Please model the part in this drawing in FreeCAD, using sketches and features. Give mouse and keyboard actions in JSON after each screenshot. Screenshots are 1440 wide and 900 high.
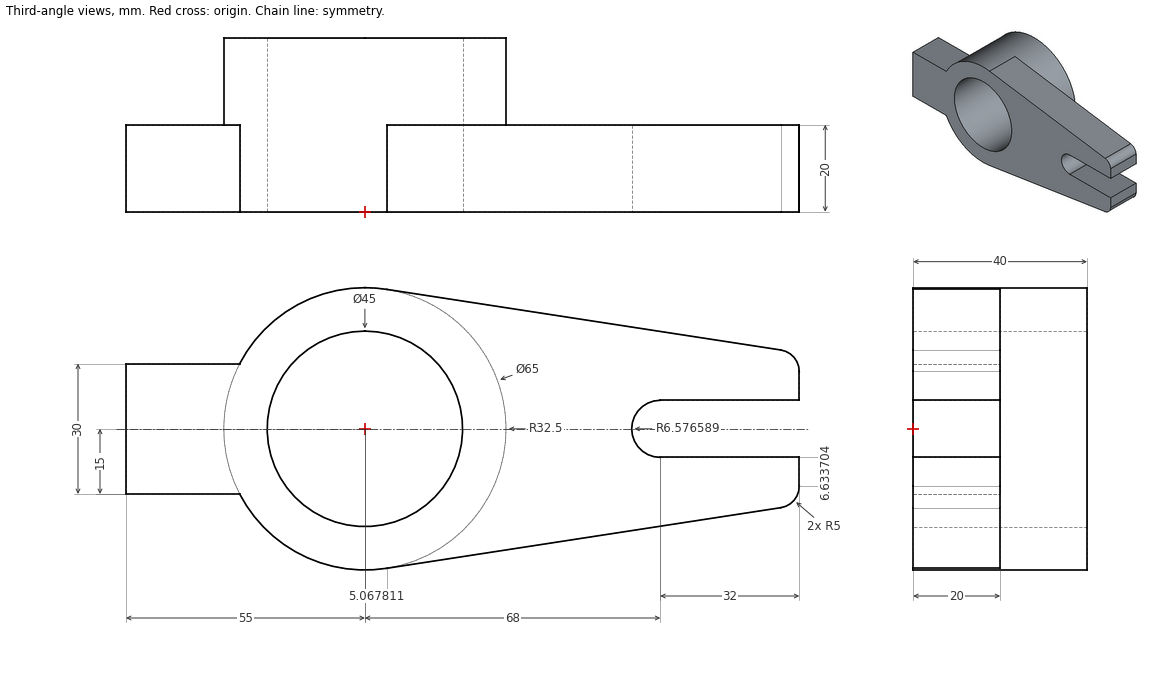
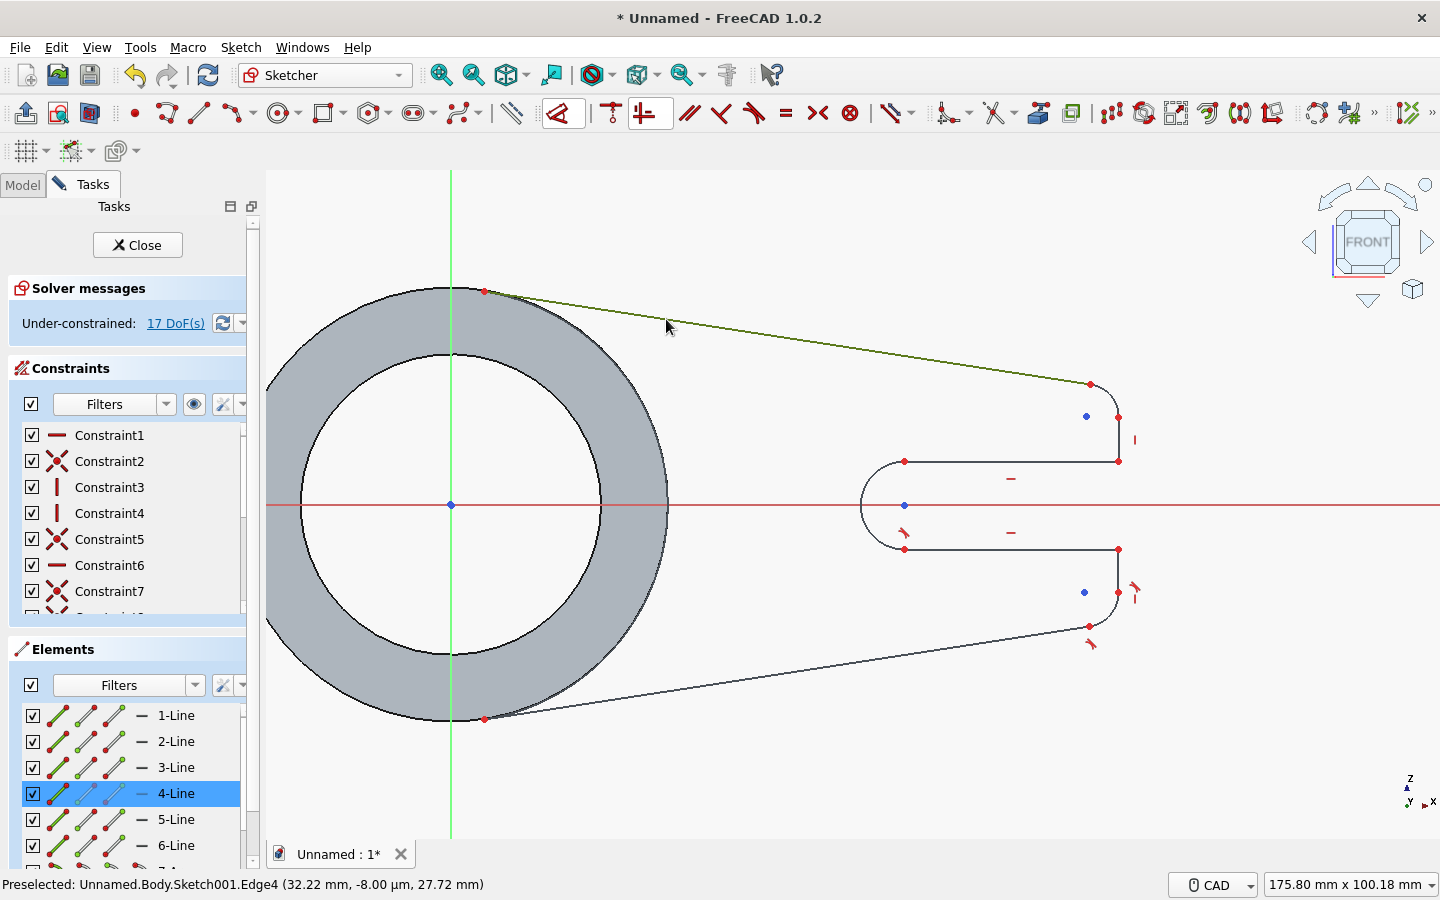
{"action": "left_click", "coordinate": [1116, 404]}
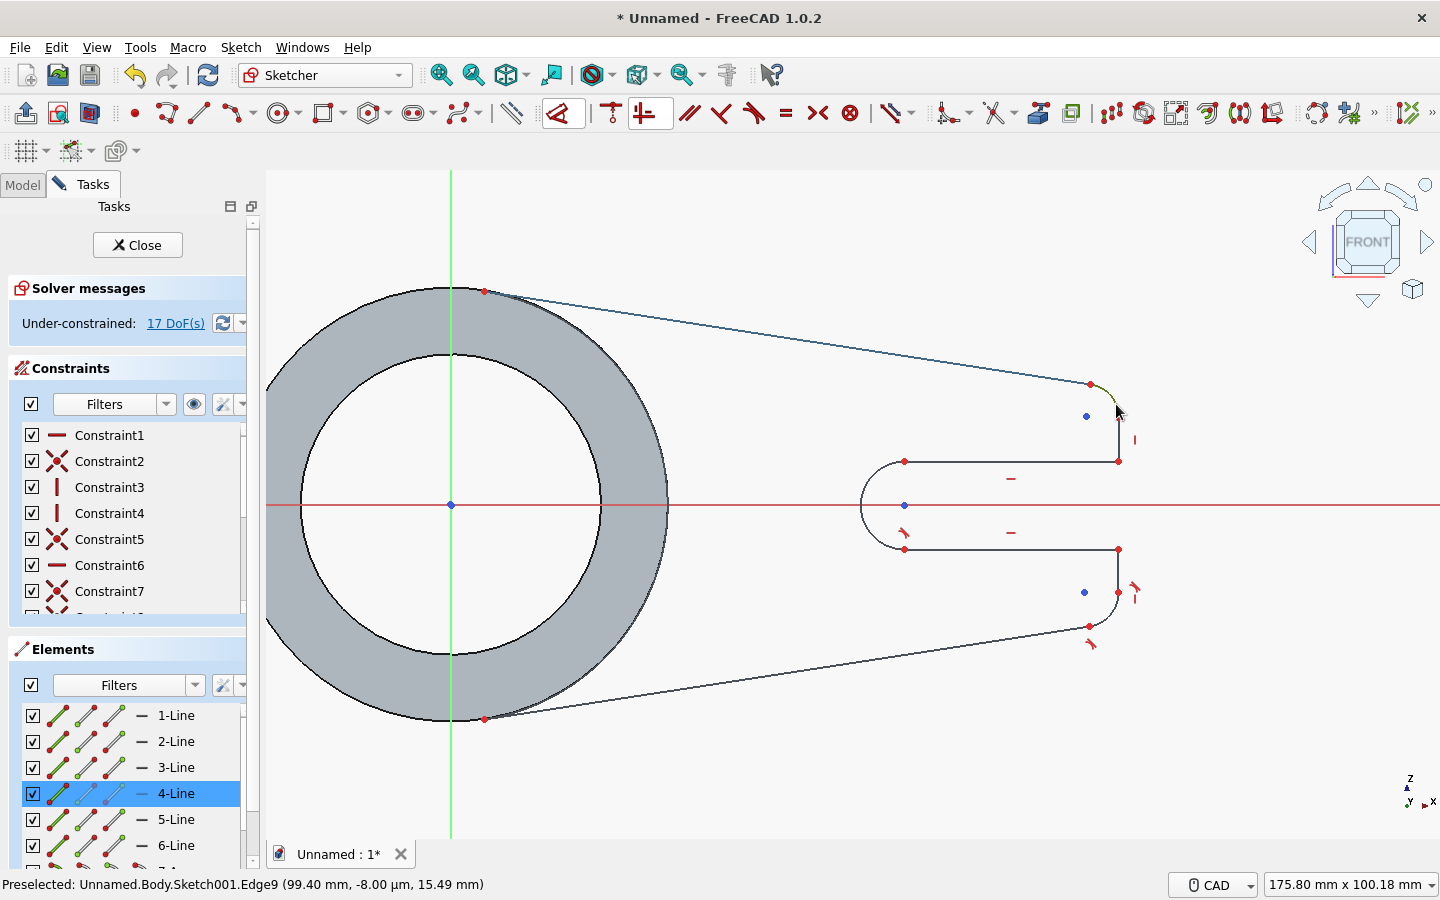
{"action": "left_click", "coordinate": [754, 114]}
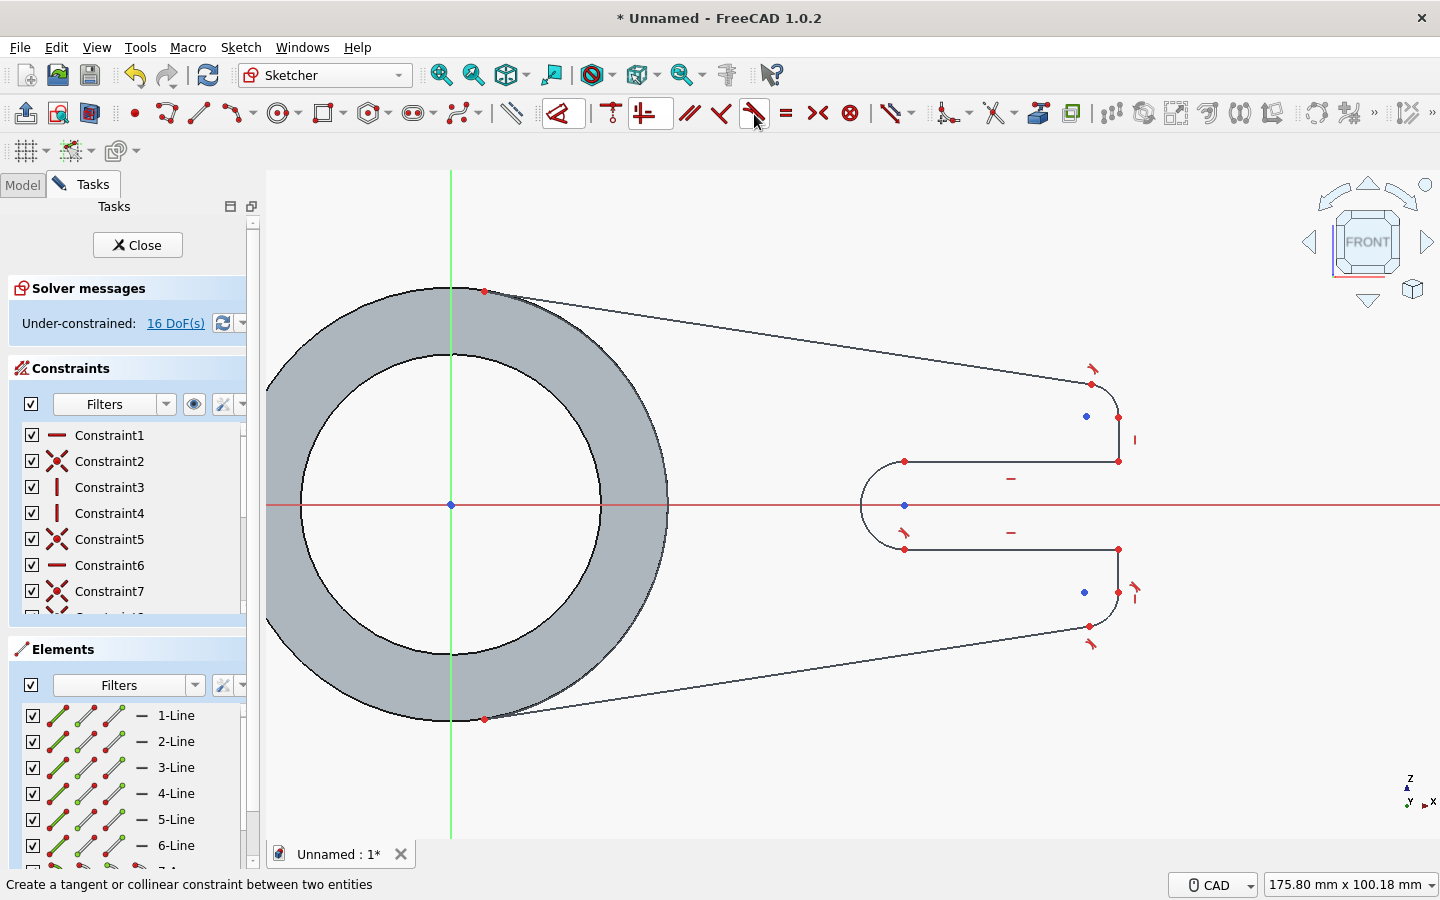
{"action": "left_click", "coordinate": [1119, 431]}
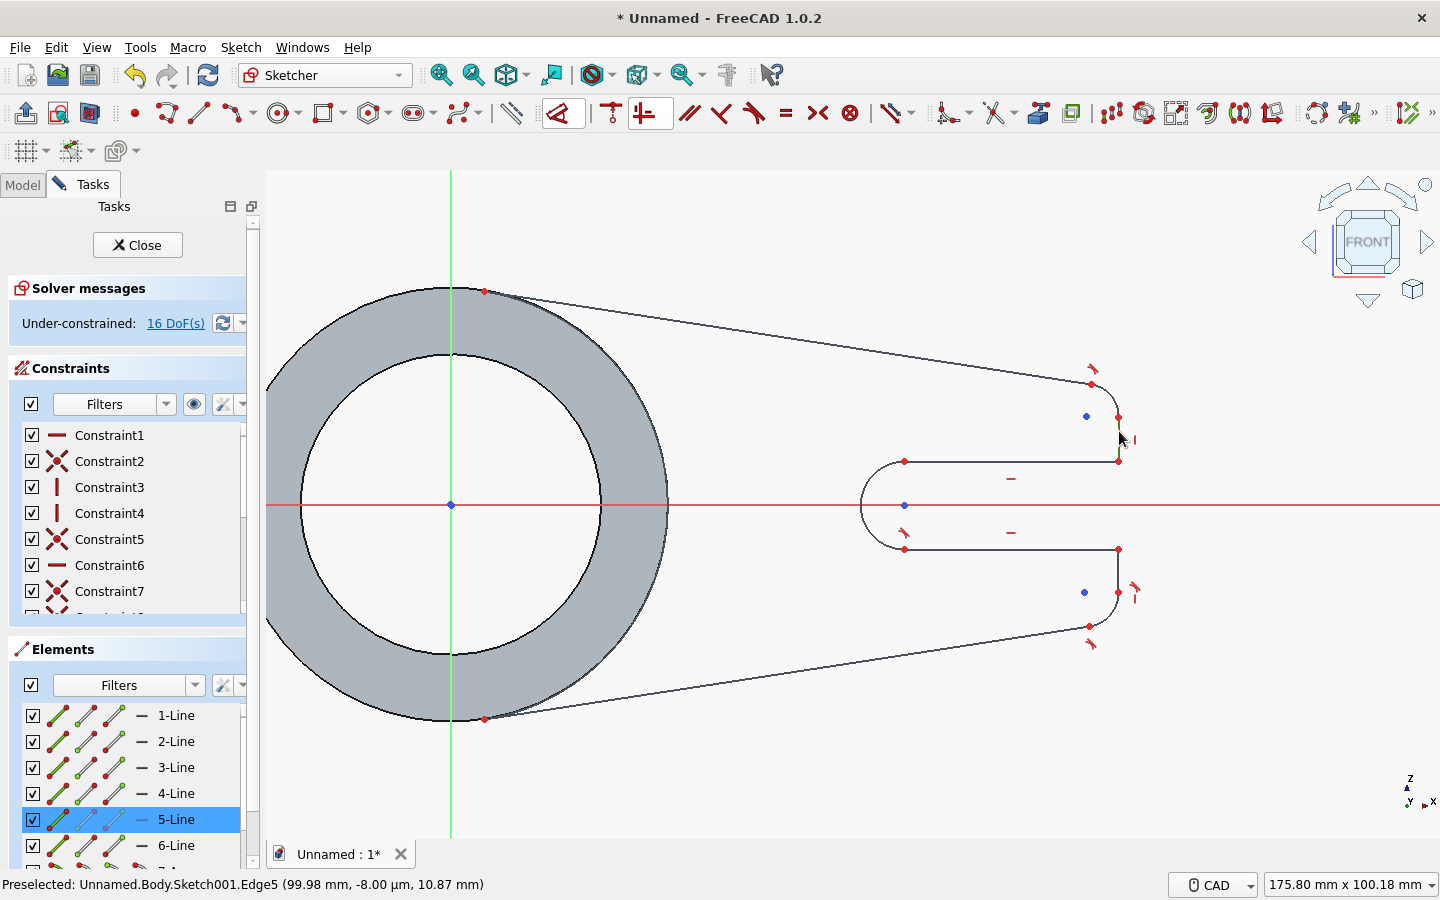
{"action": "left_click", "coordinate": [1116, 404]}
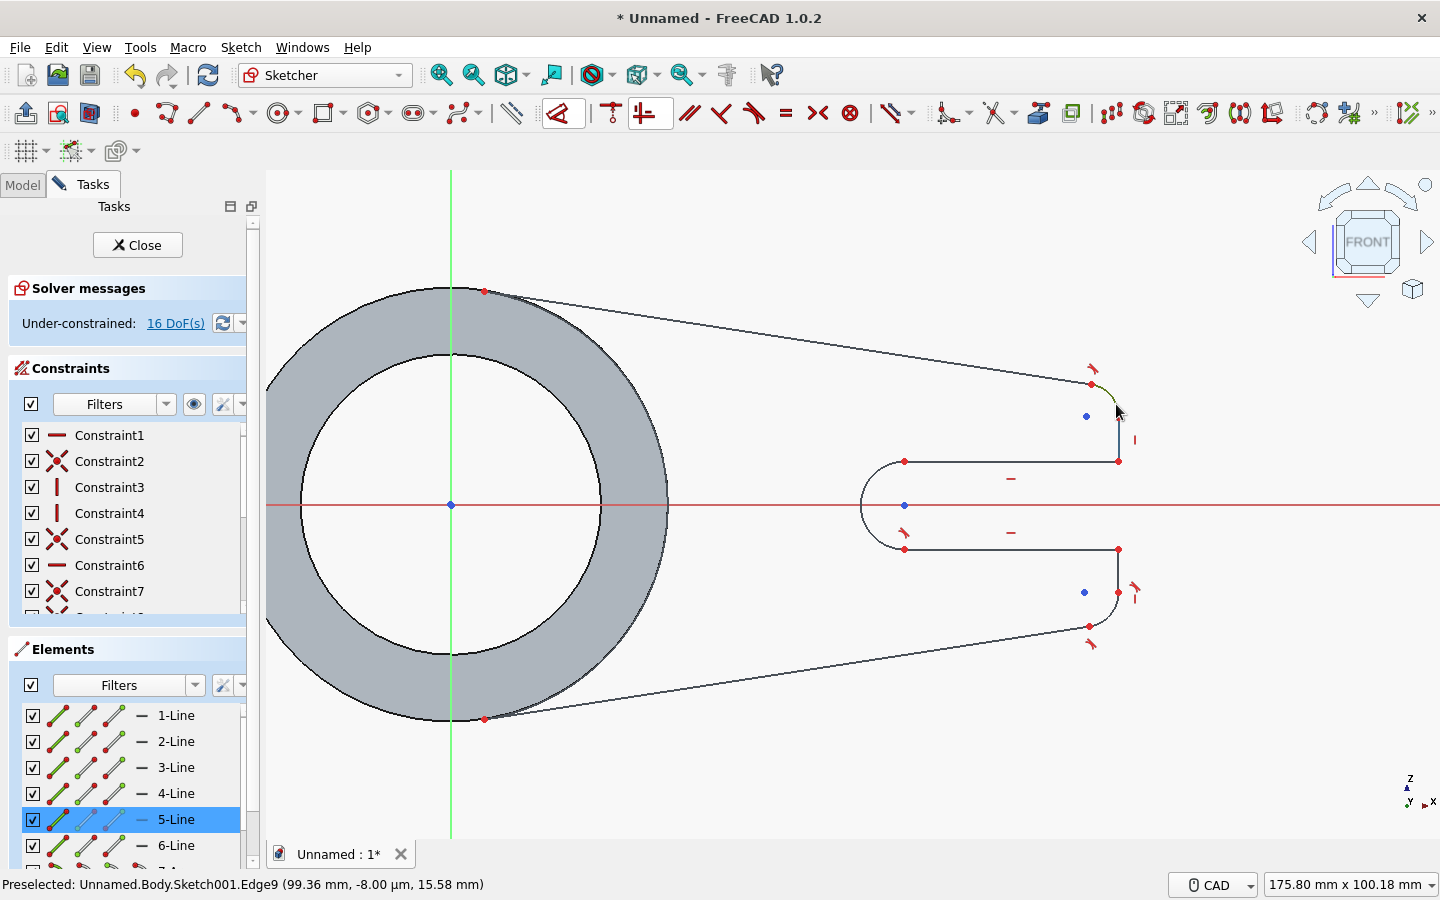
{"action": "left_click", "coordinate": [754, 114]}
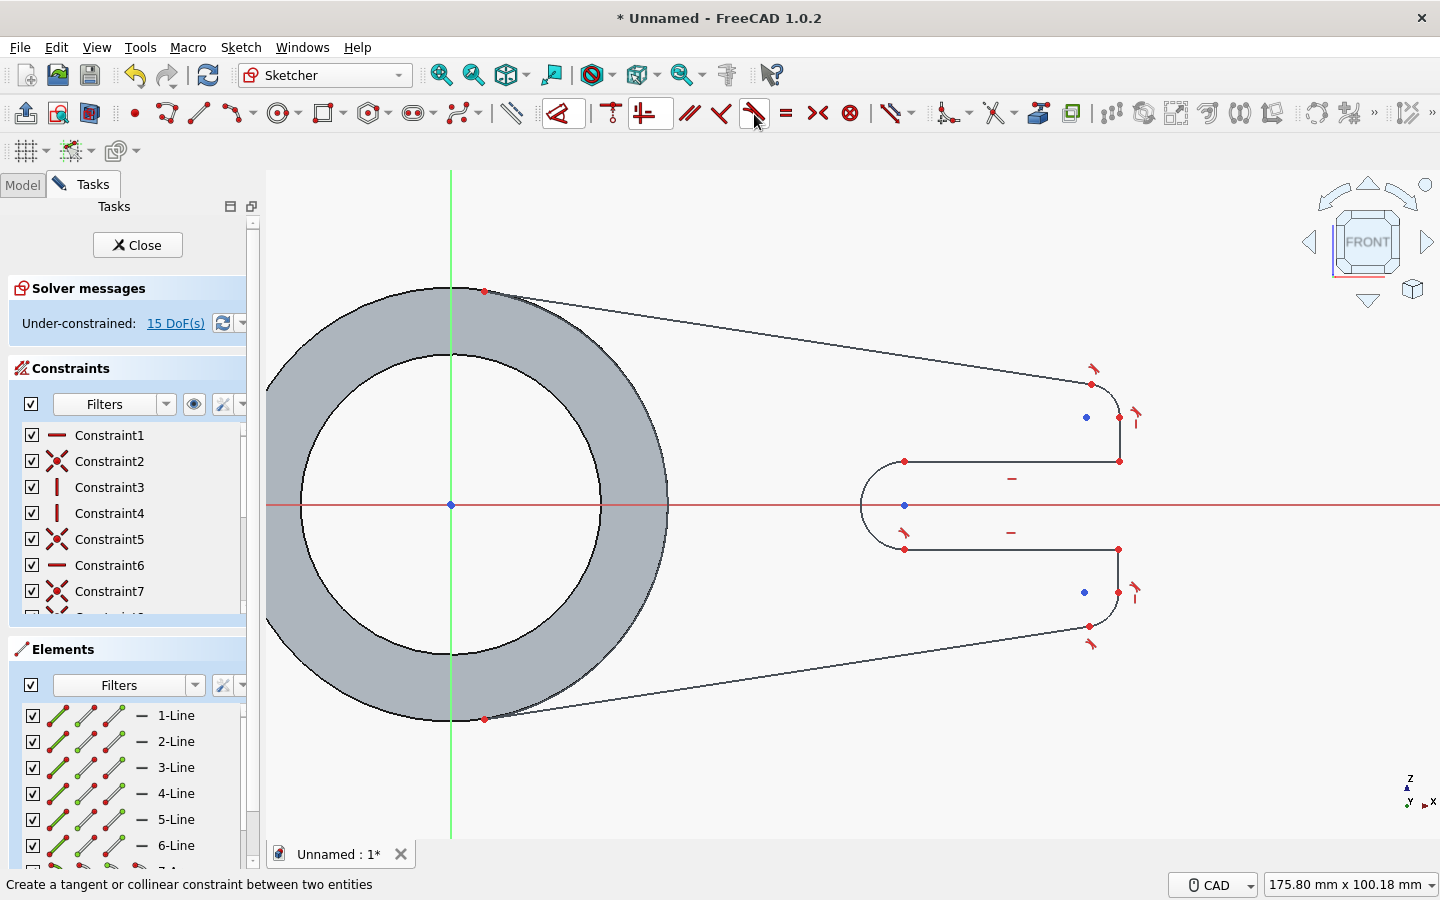
{"action": "left_click", "coordinate": [1055, 462]}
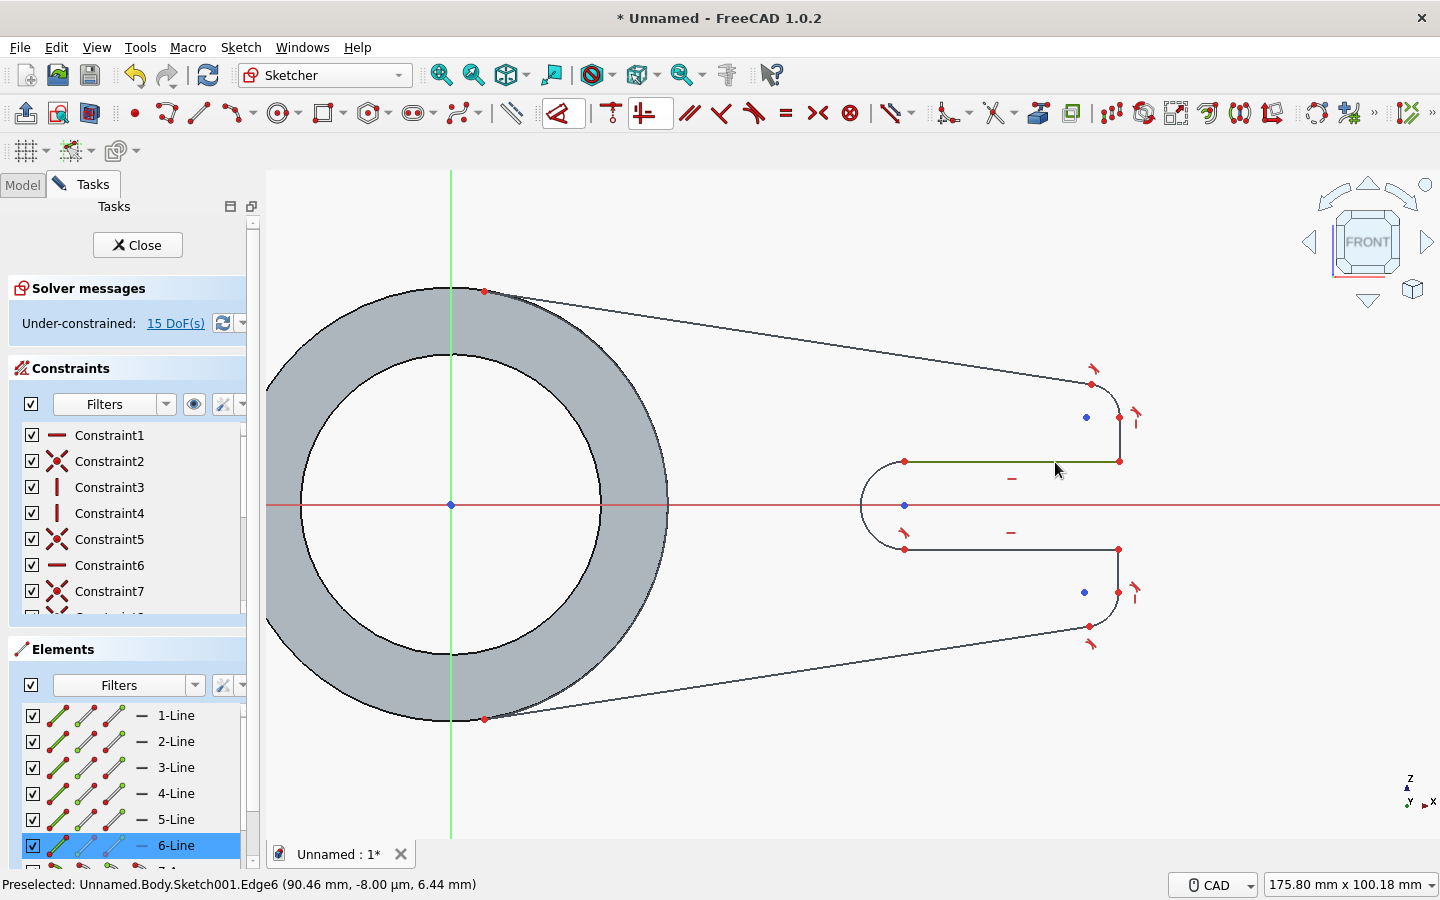
{"action": "left_click", "coordinate": [869, 480]}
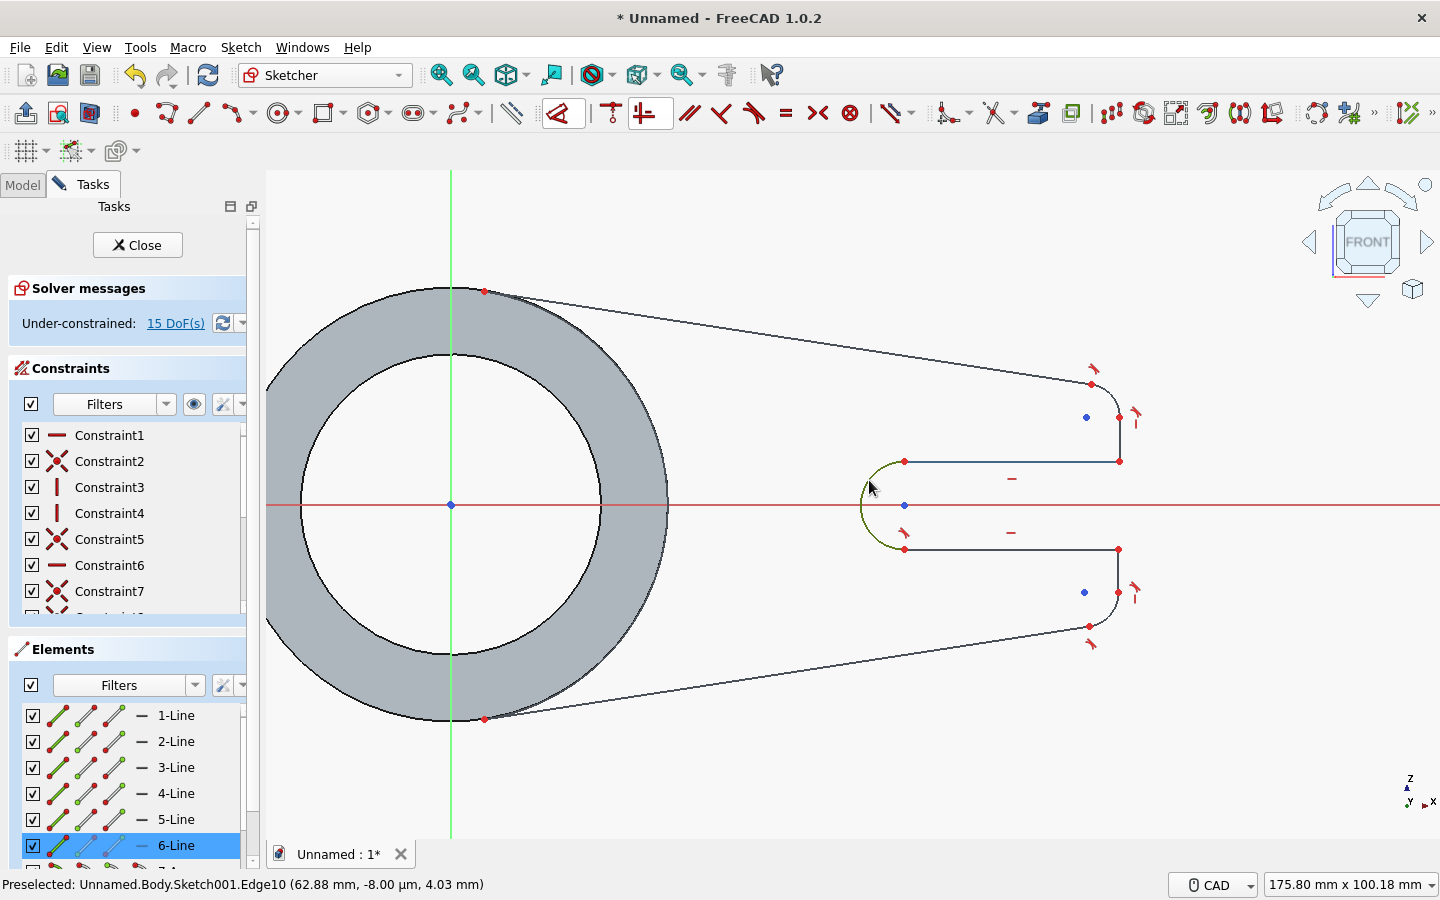
{"action": "left_click", "coordinate": [754, 114]}